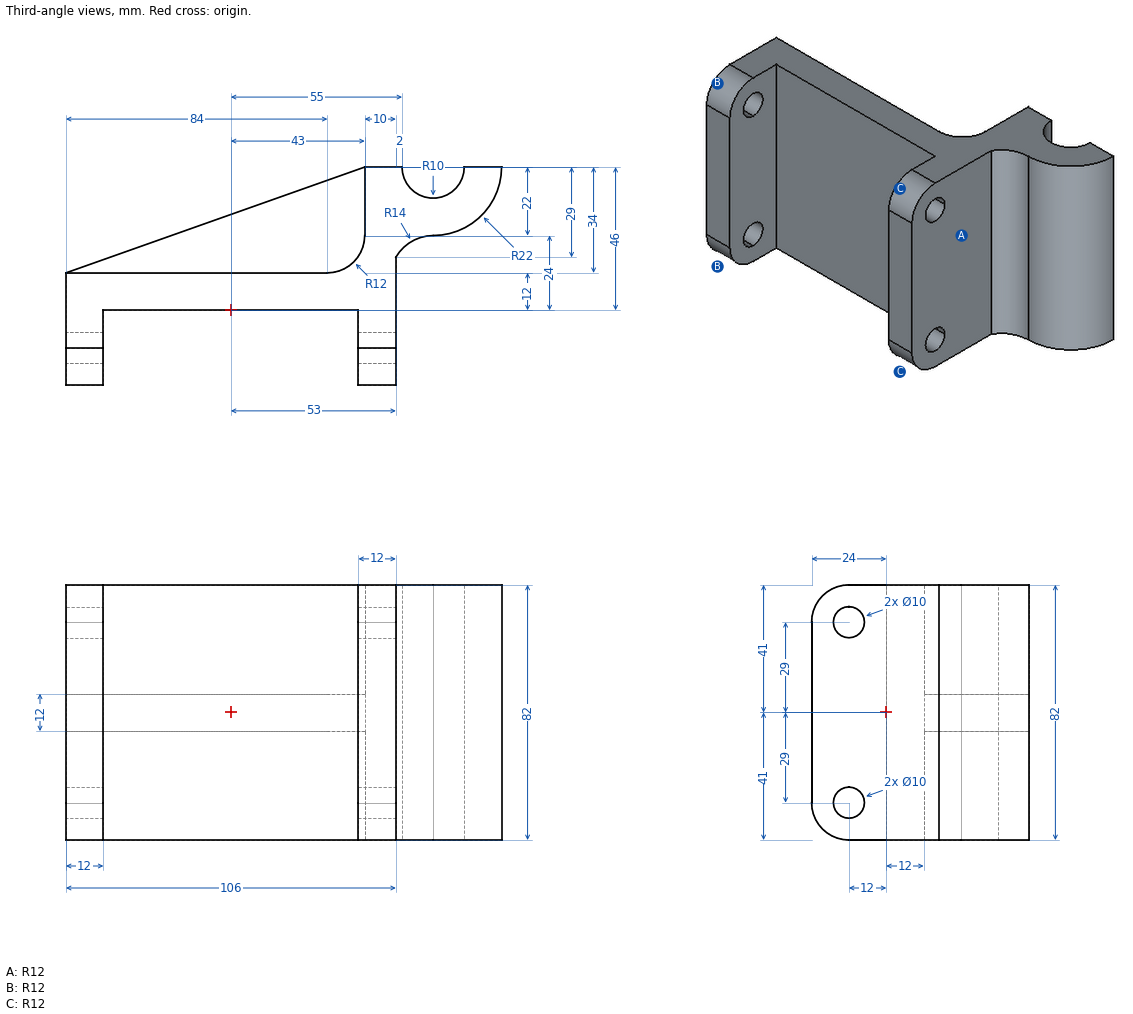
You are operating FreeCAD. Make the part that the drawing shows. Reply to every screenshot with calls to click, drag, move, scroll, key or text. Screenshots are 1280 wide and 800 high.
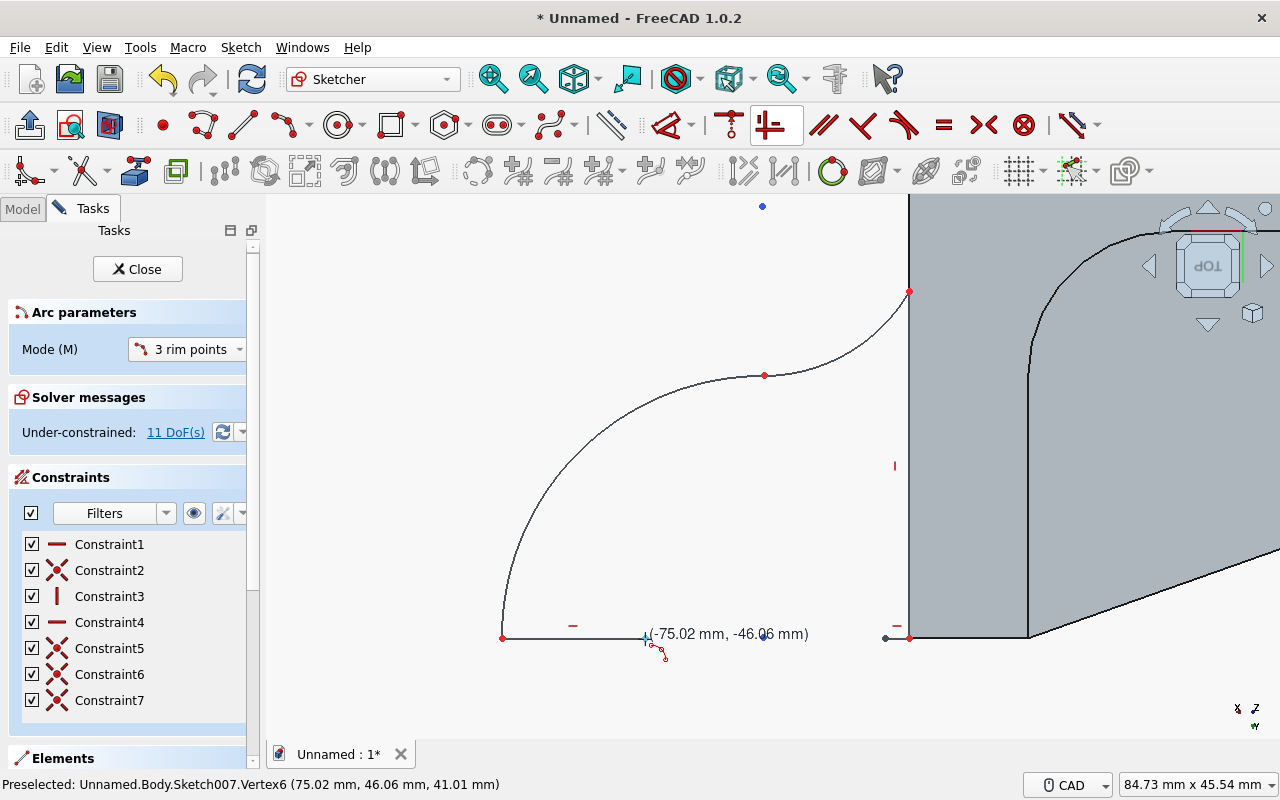
scroll(885, 638, up, 2)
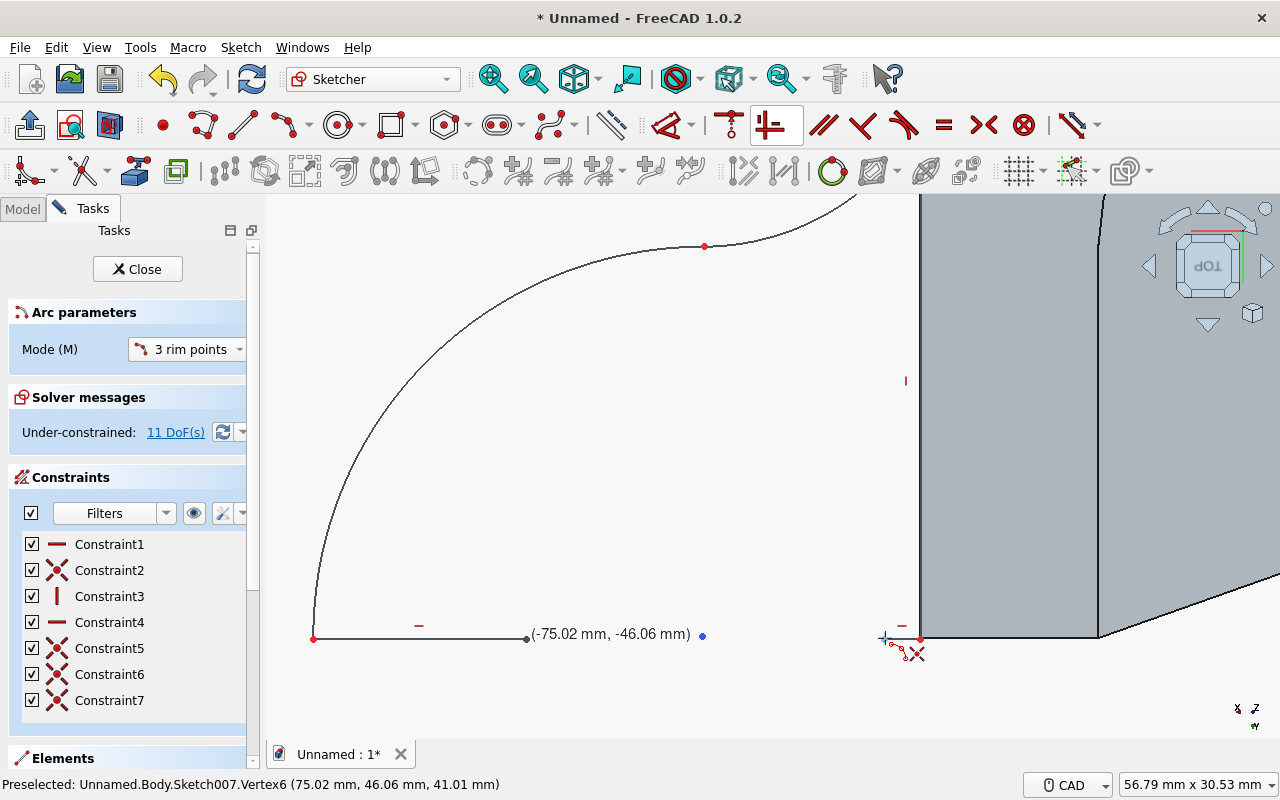
click(885, 639)
click(706, 460)
key(Escape)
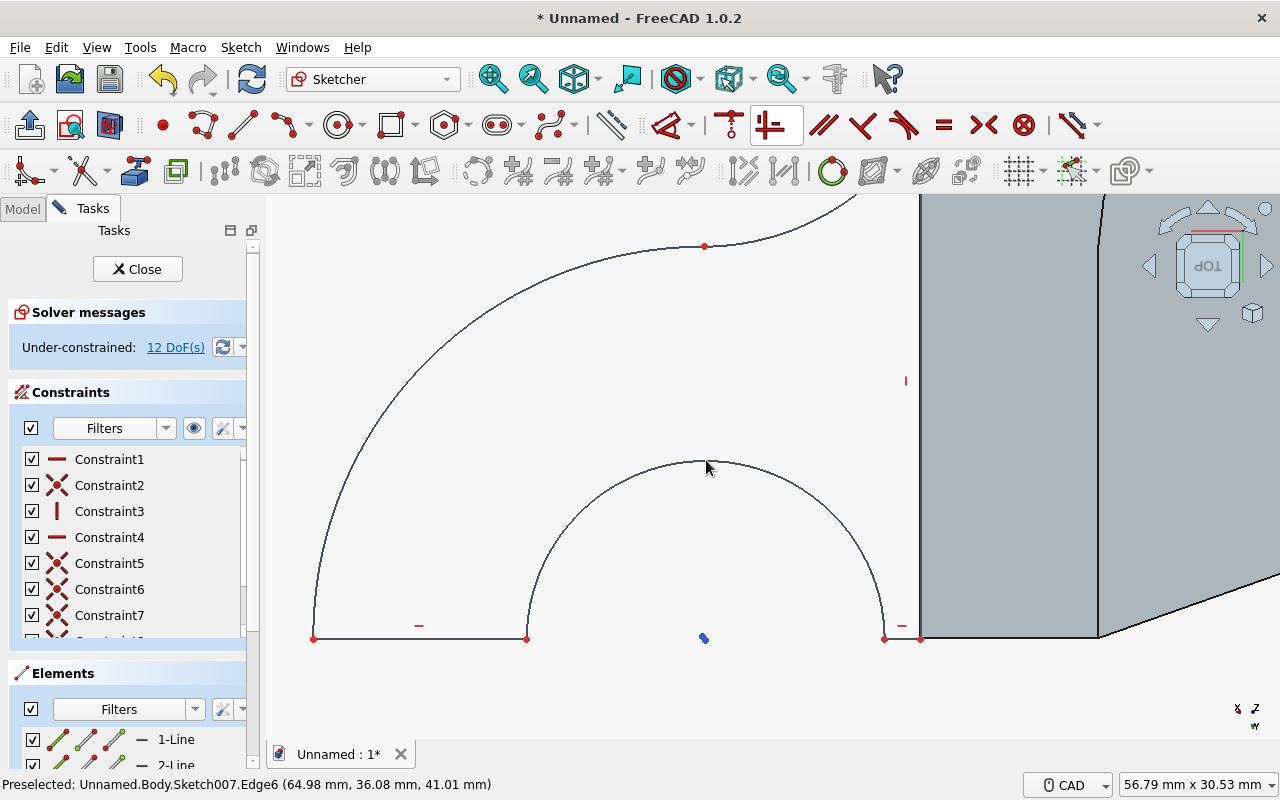
click(781, 234)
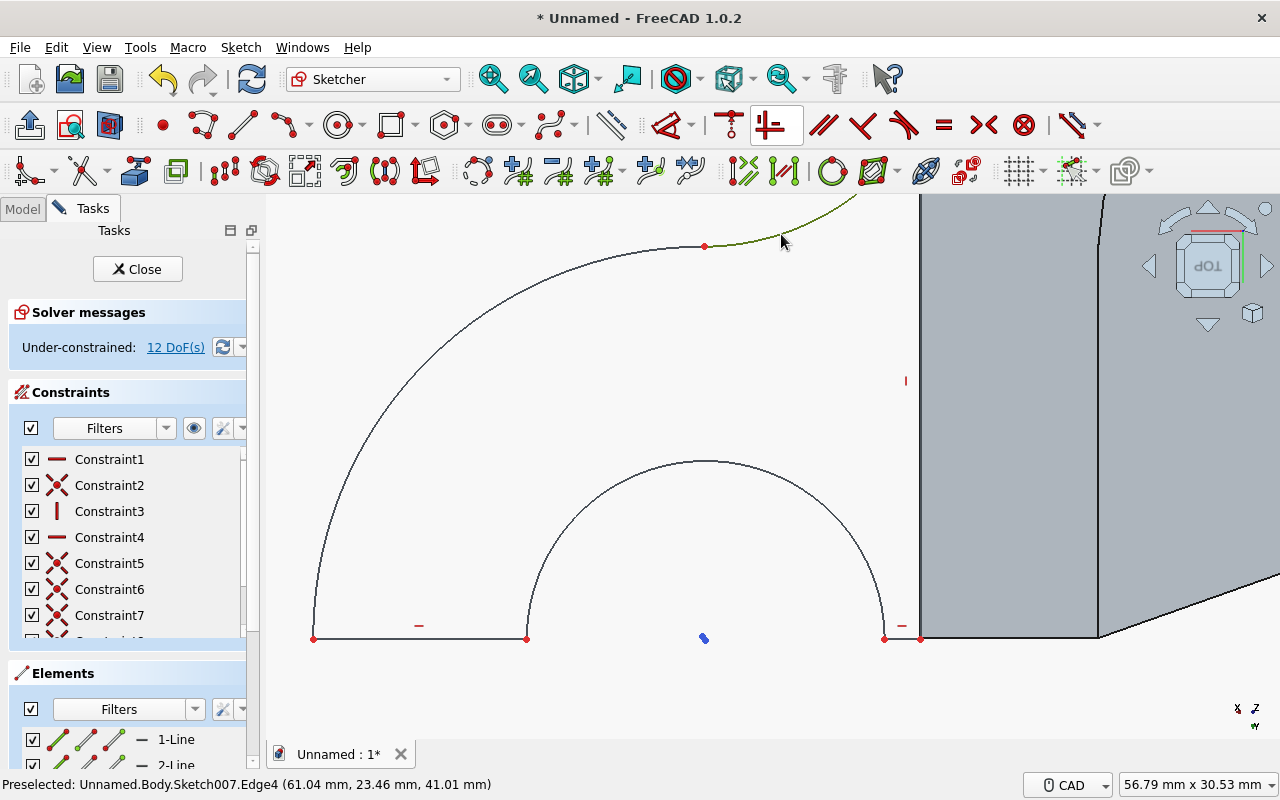
click(526, 289)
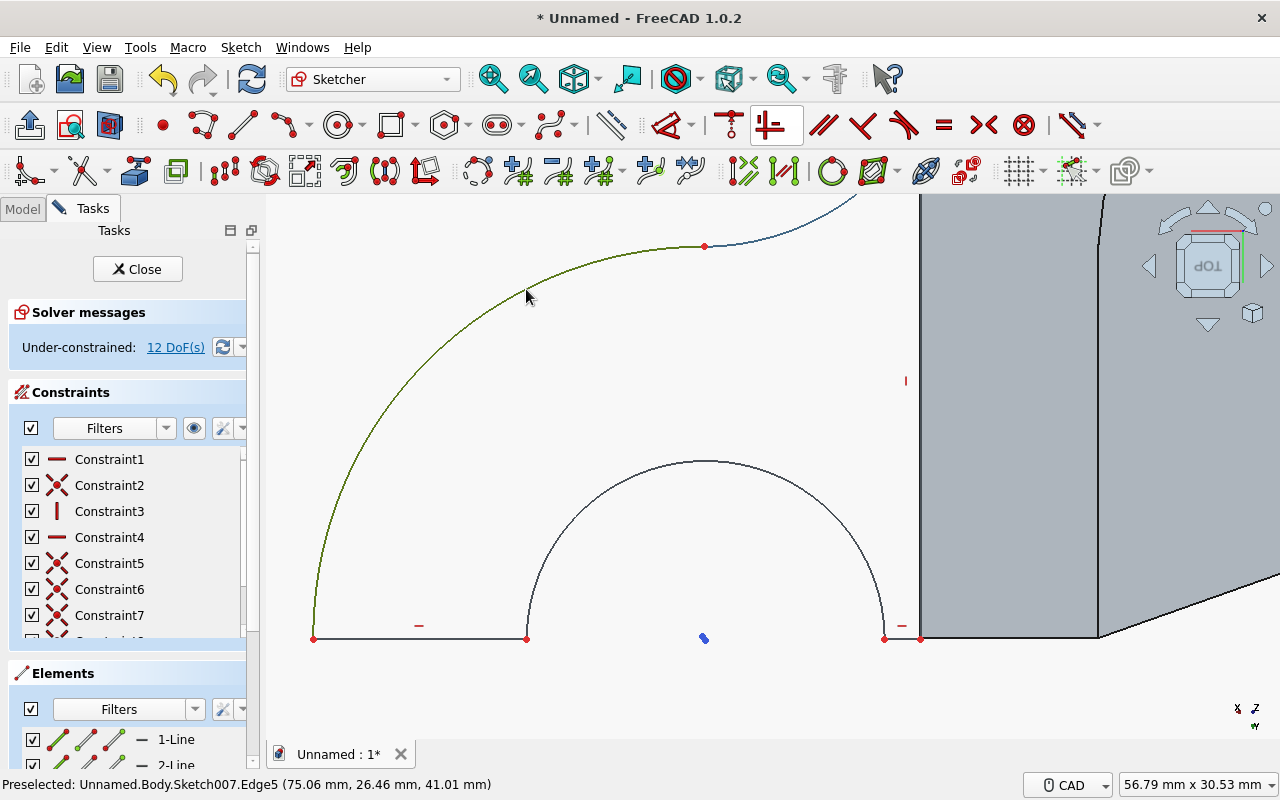
key(t)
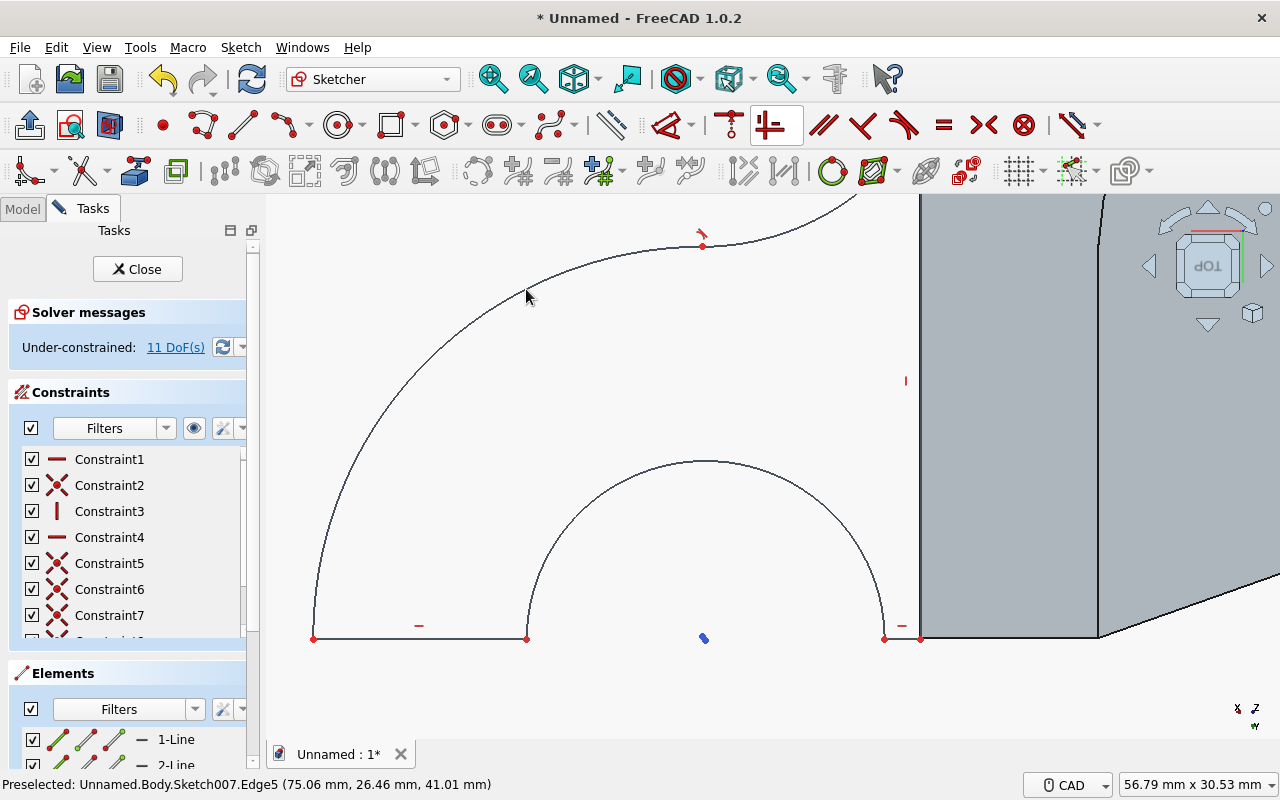
click(525, 290)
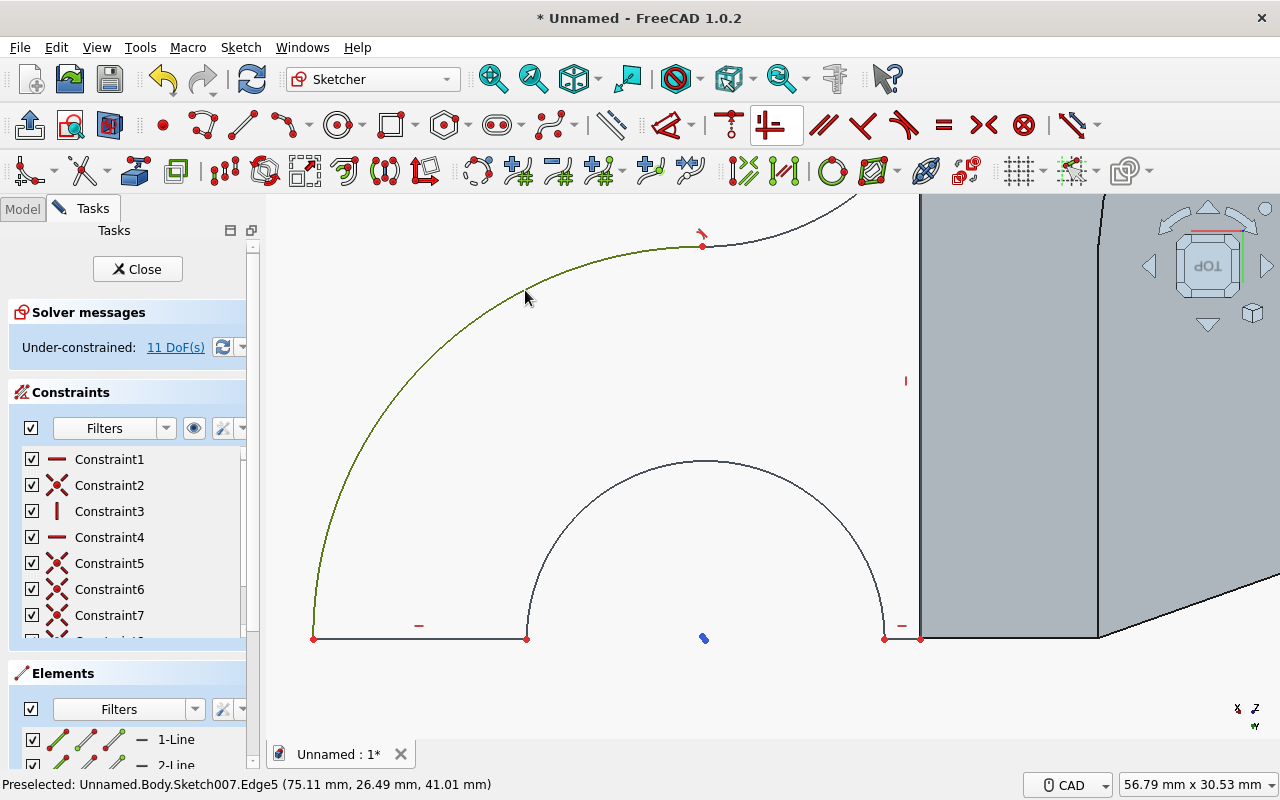
click(811, 495)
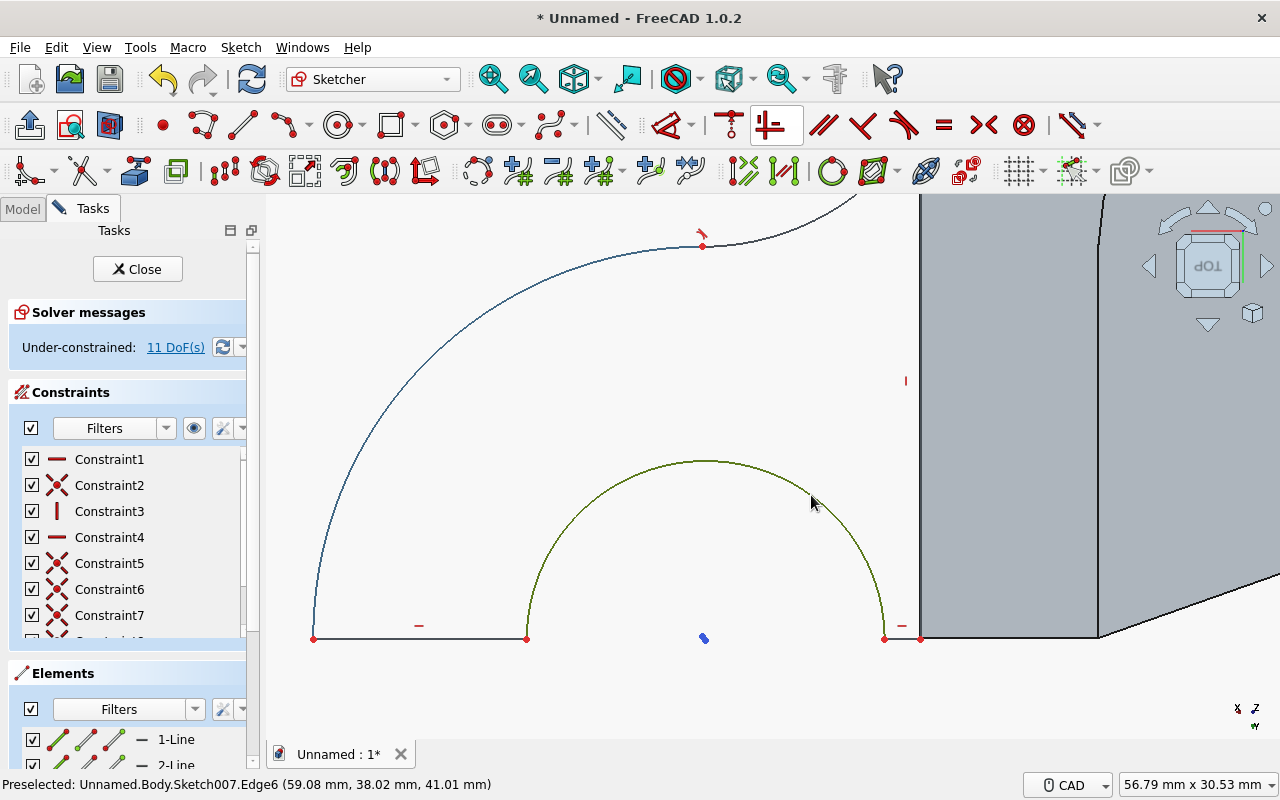
key(c)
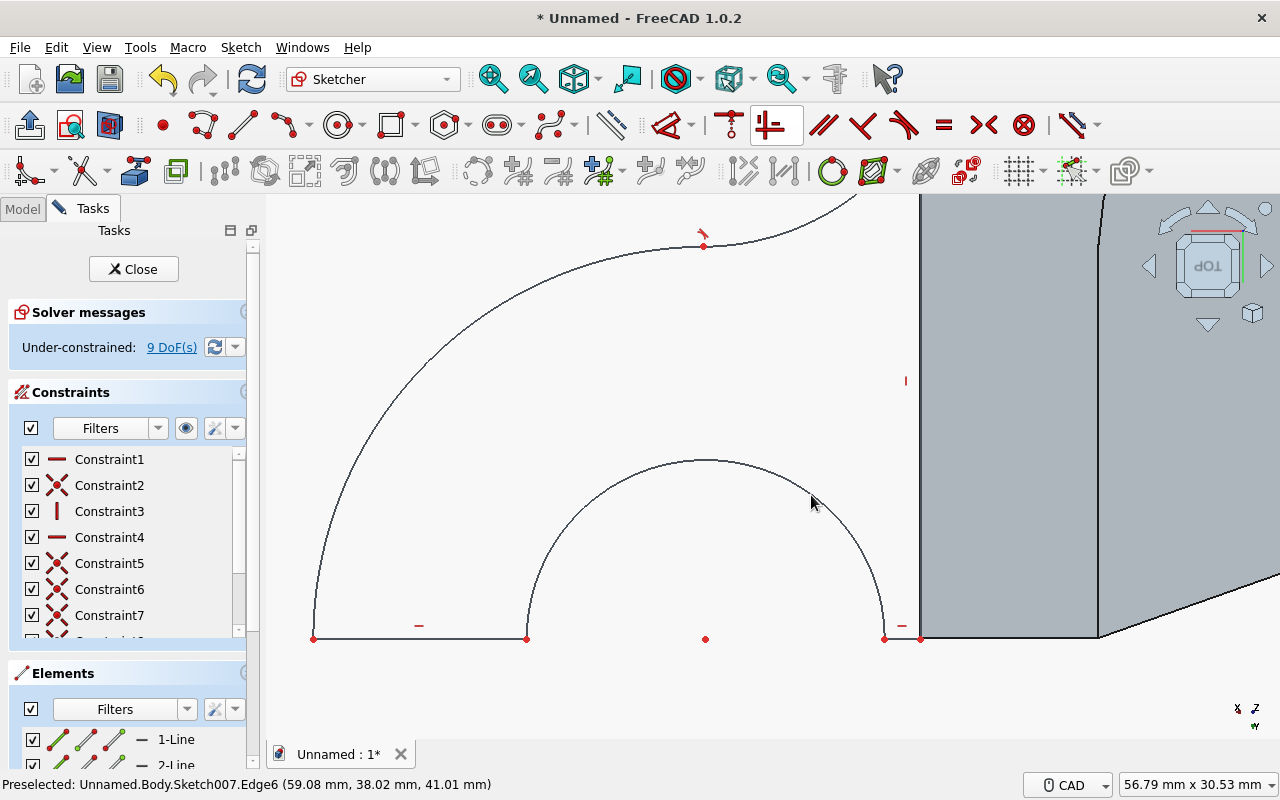
key(d)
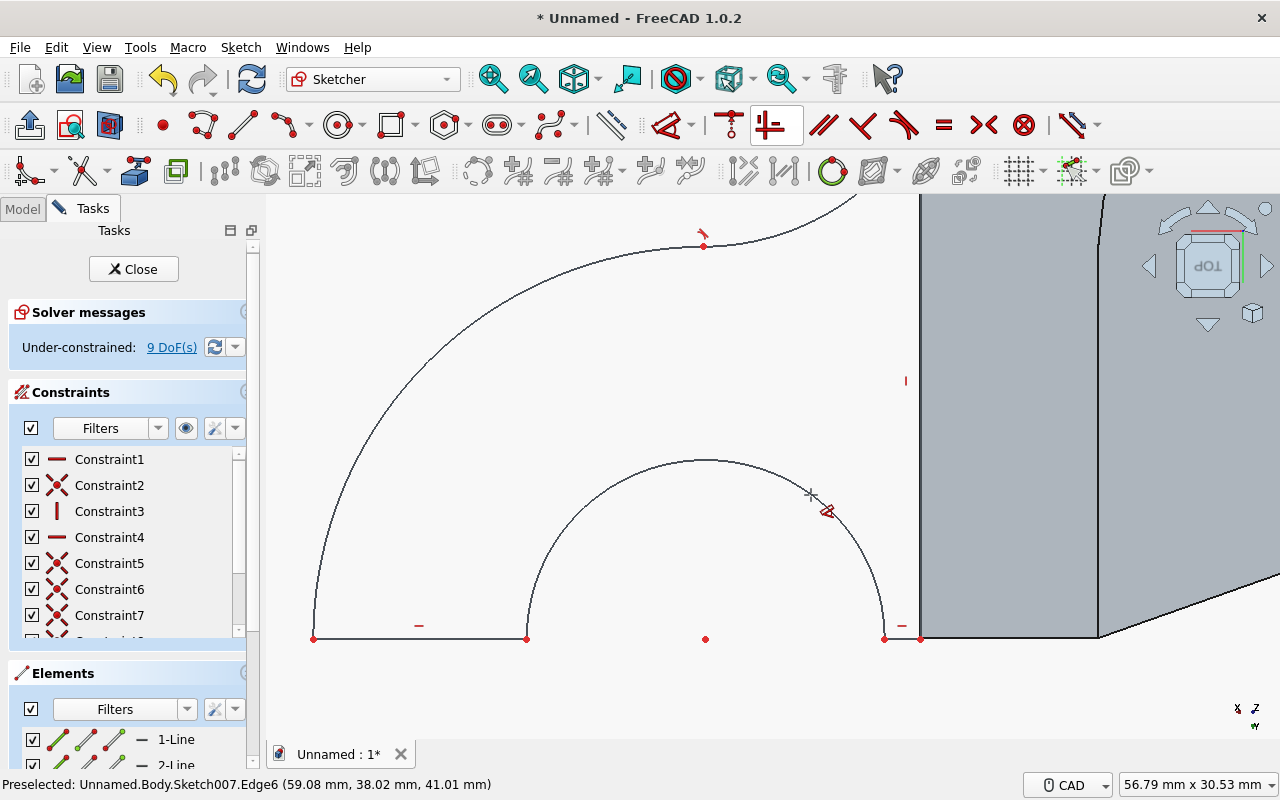
click(781, 234)
click(791, 264)